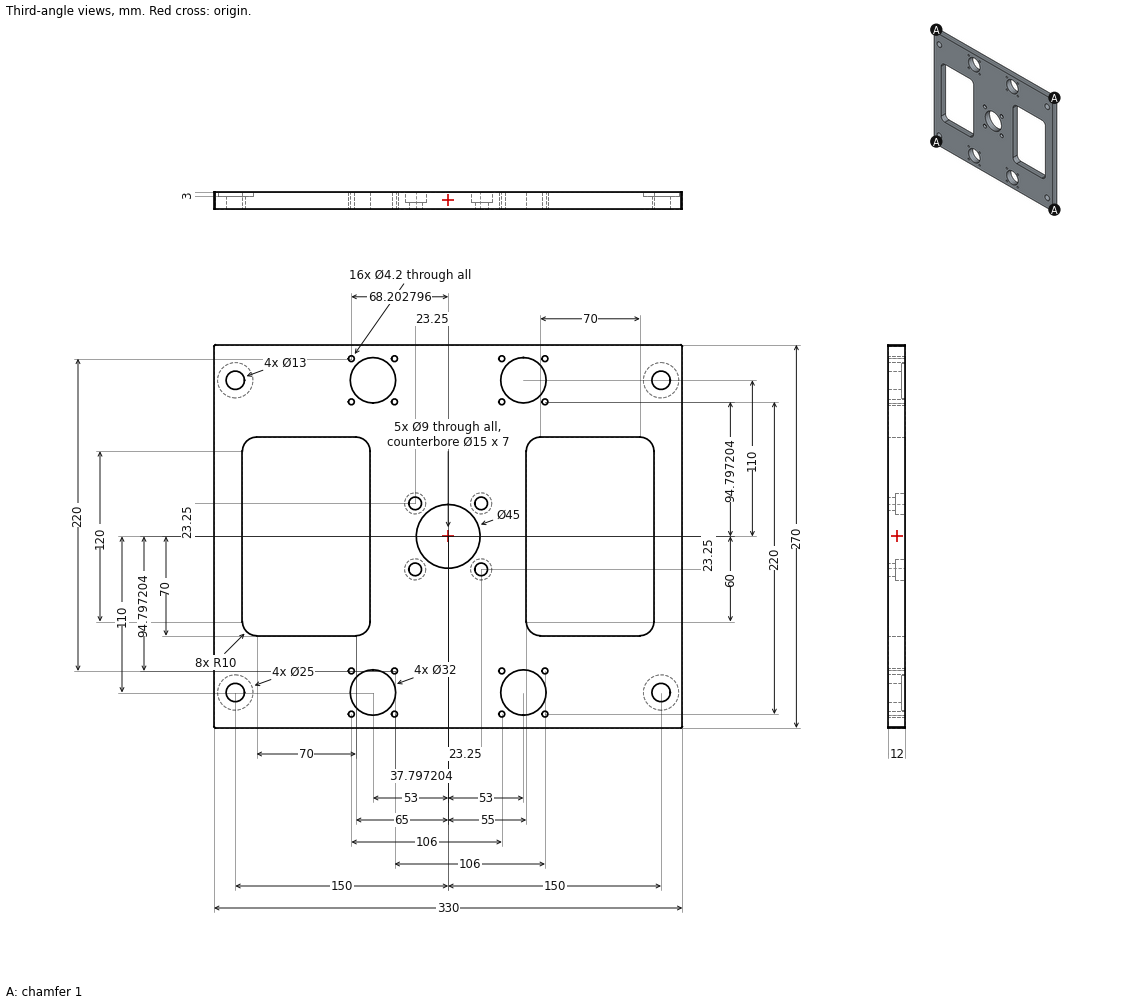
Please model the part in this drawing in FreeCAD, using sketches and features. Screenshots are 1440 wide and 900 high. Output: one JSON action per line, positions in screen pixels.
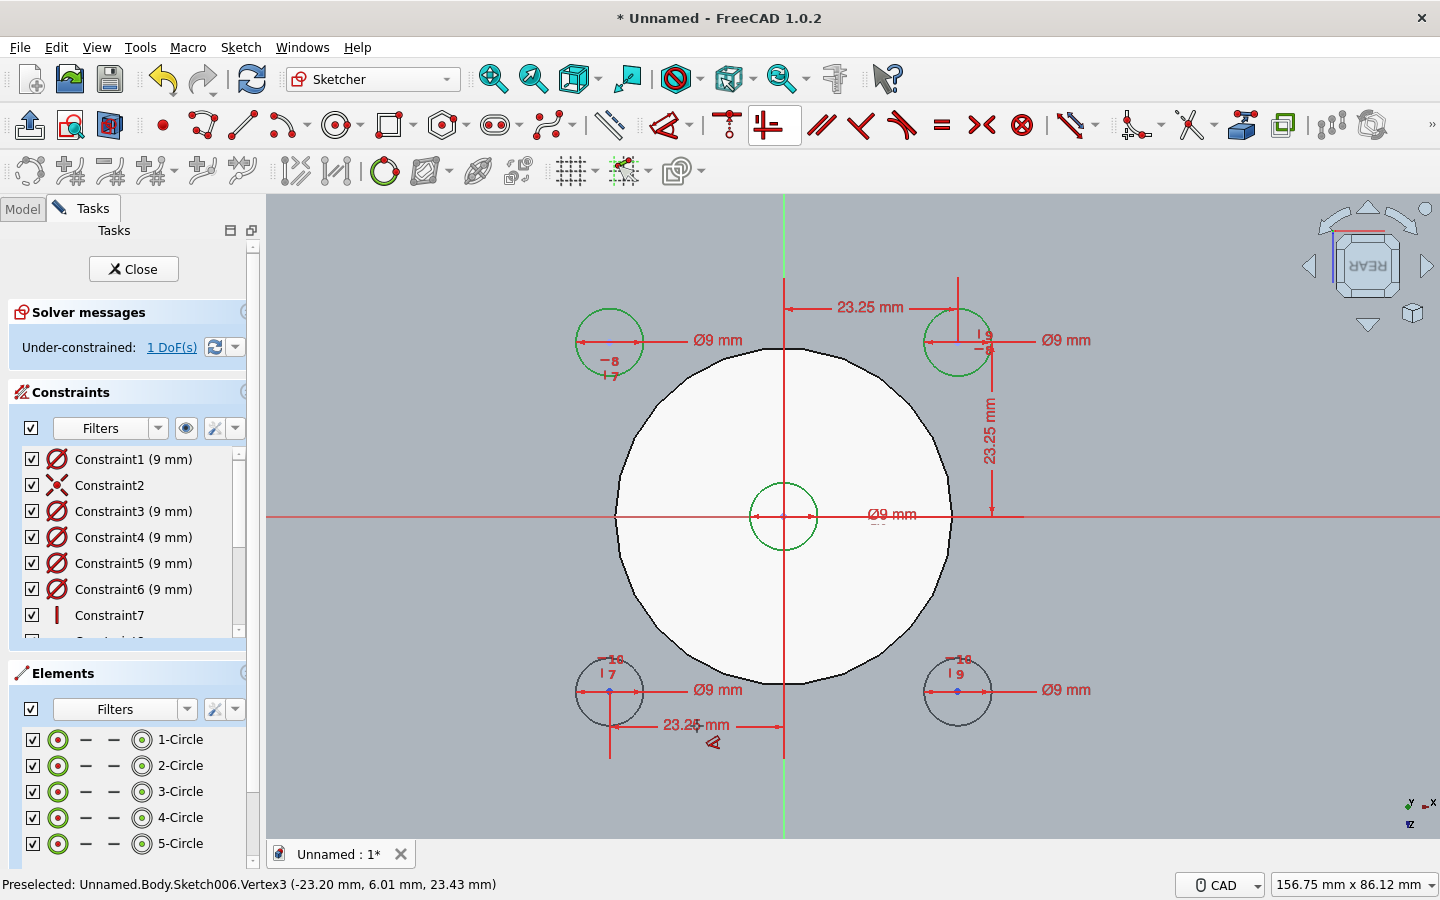
{"action": "left_click", "coordinate": [610, 692]}
{"action": "left_click", "coordinate": [576, 604]}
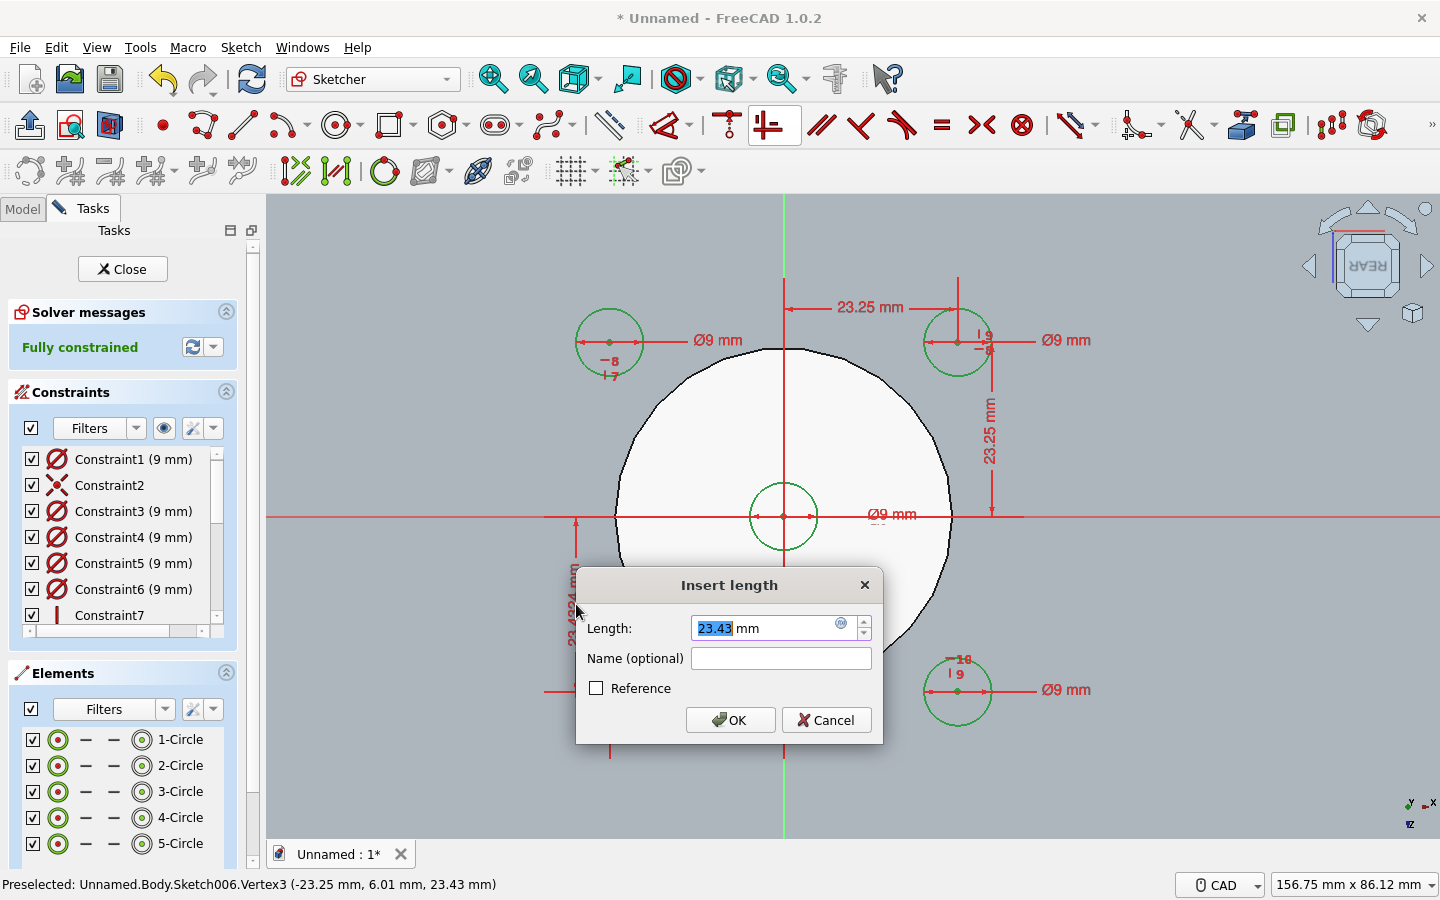
{"action": "type", "text": "23.25"}
{"action": "key", "text": "Return"}
{"action": "key", "text": "Escape"}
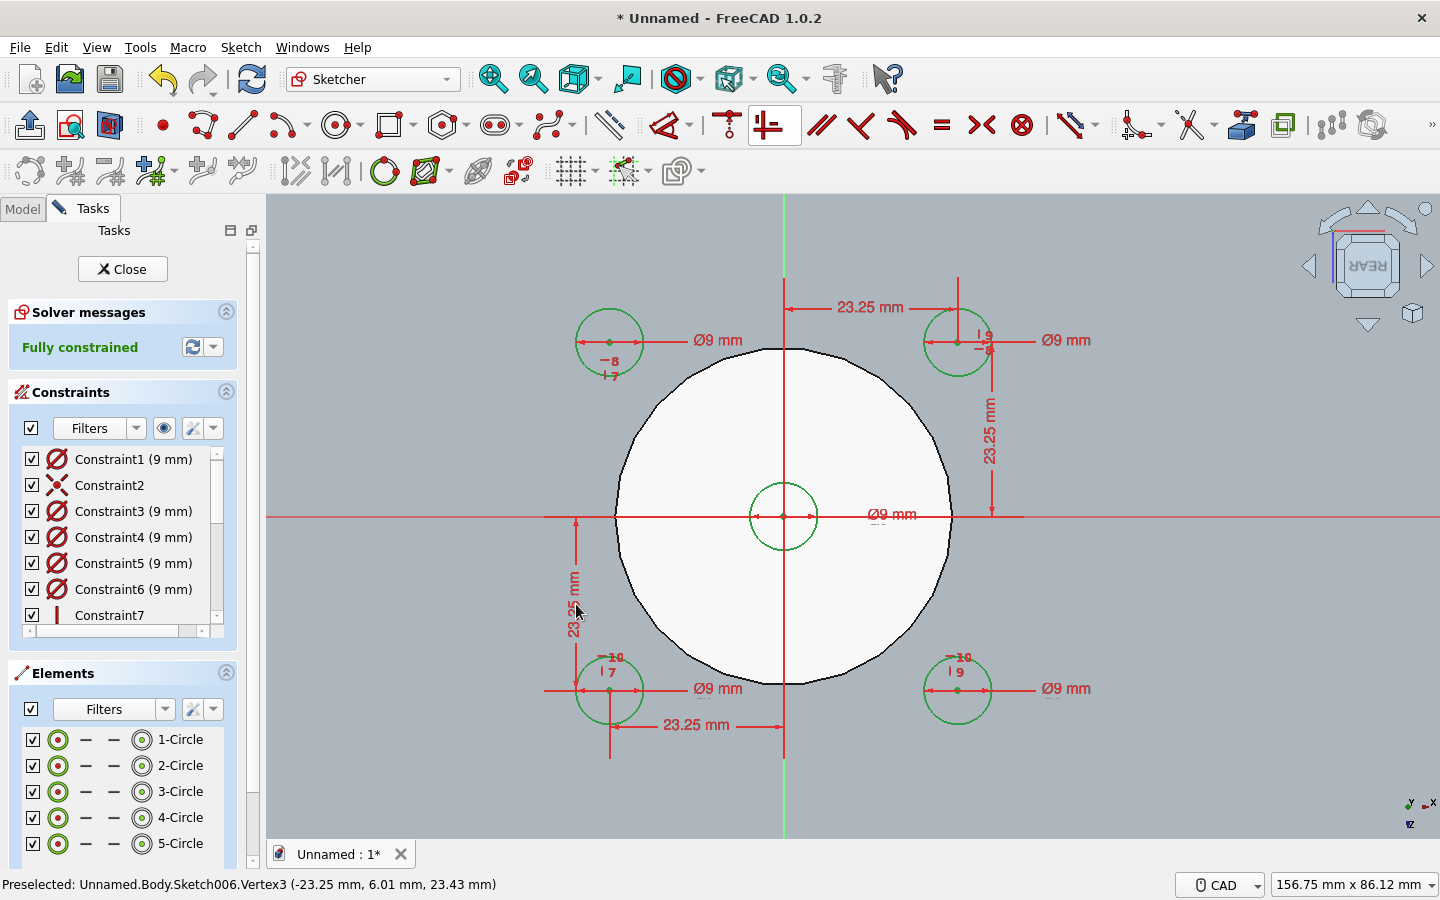
{"action": "left_click", "coordinate": [123, 269]}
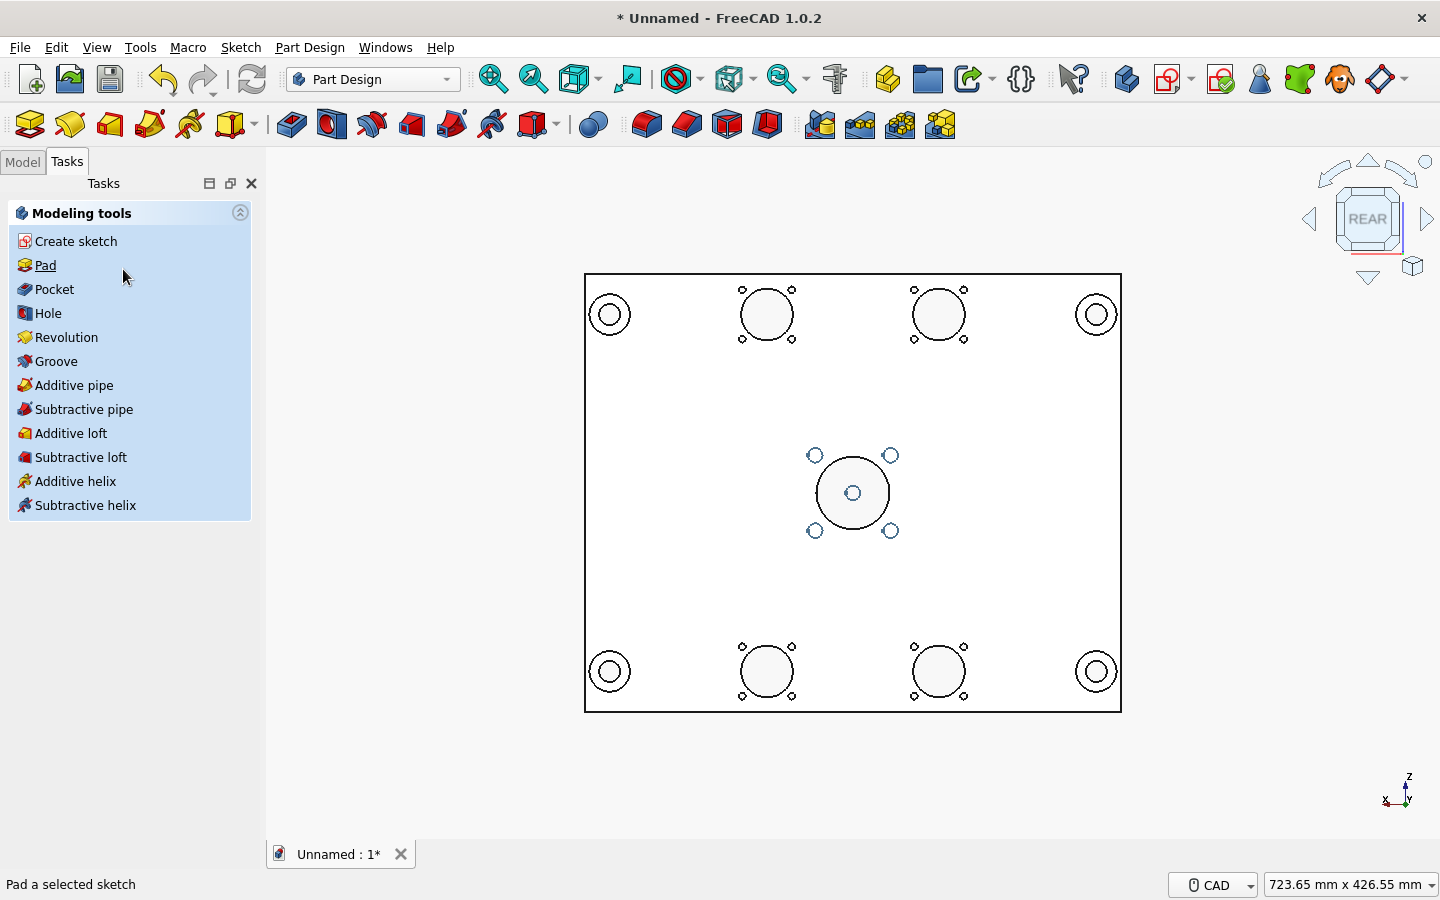
{"action": "left_click", "coordinate": [332, 124]}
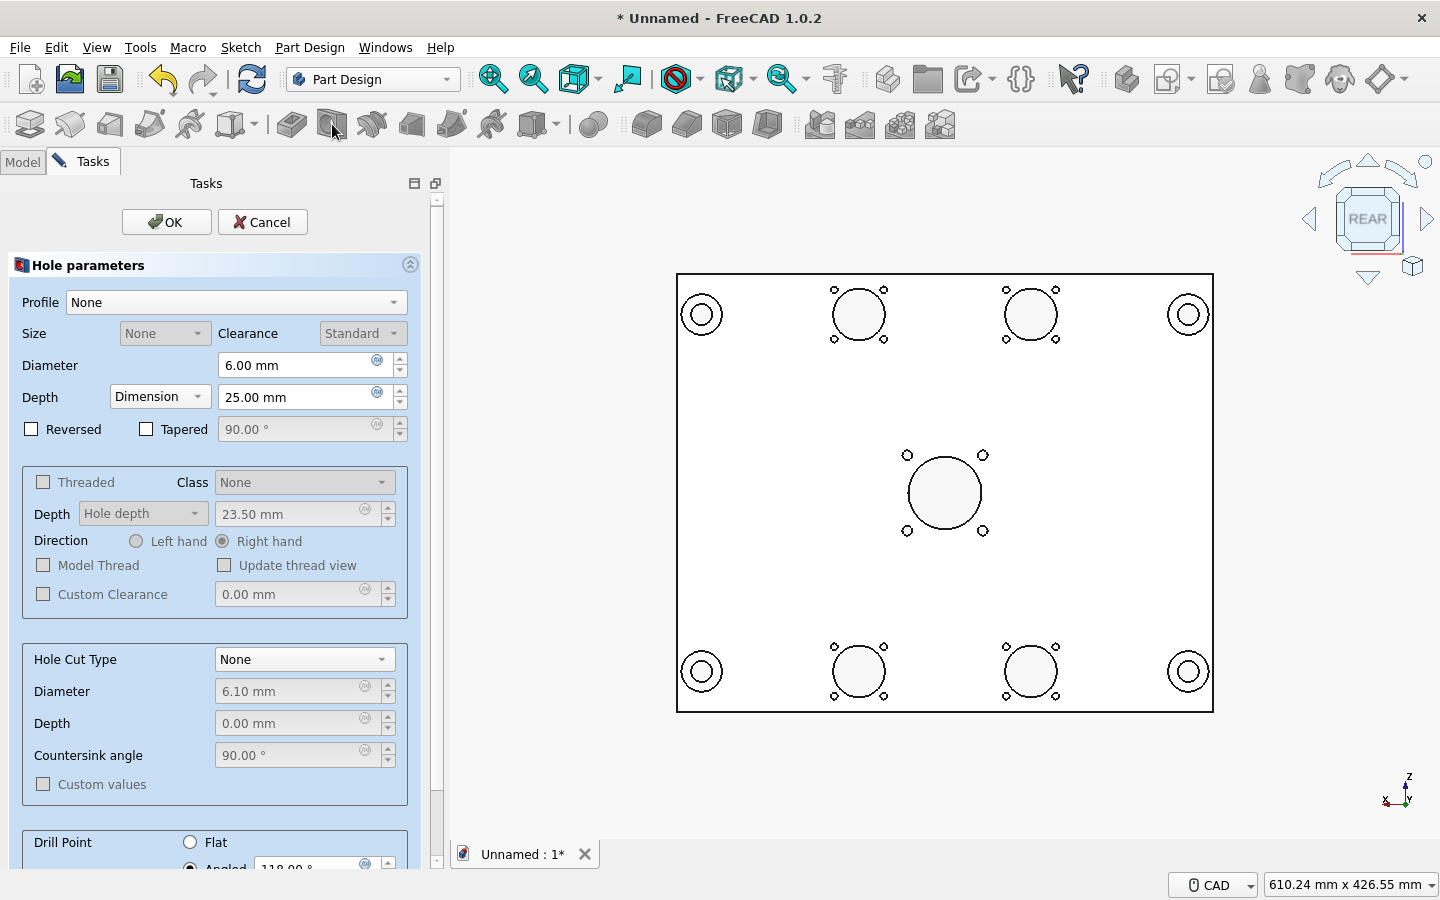
{"action": "triple_click", "coordinate": [305, 365]}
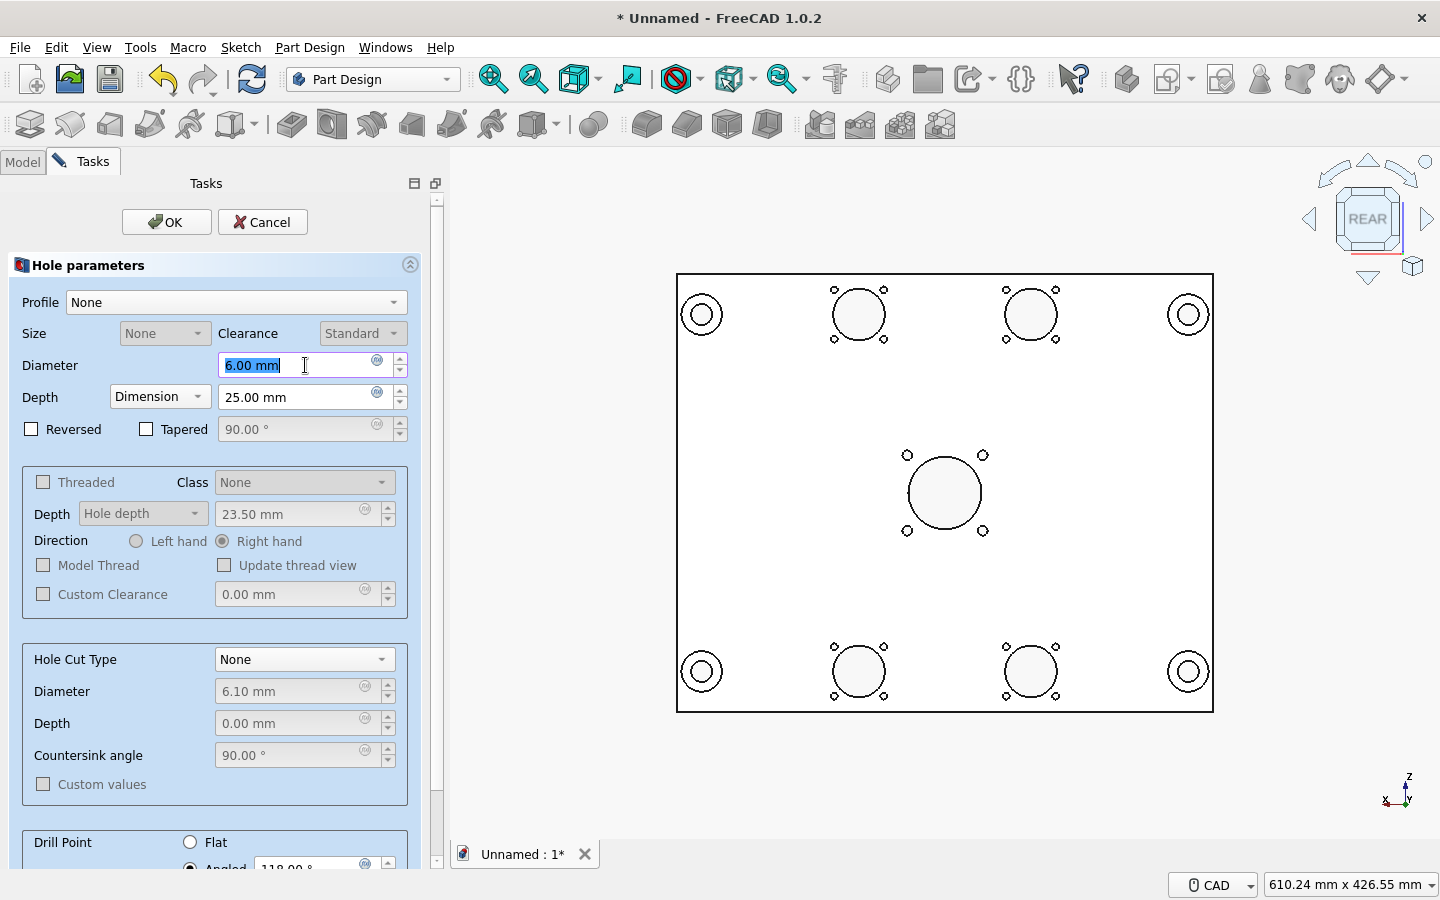
{"action": "type", "text": "9"}
{"action": "key", "text": "Tab"}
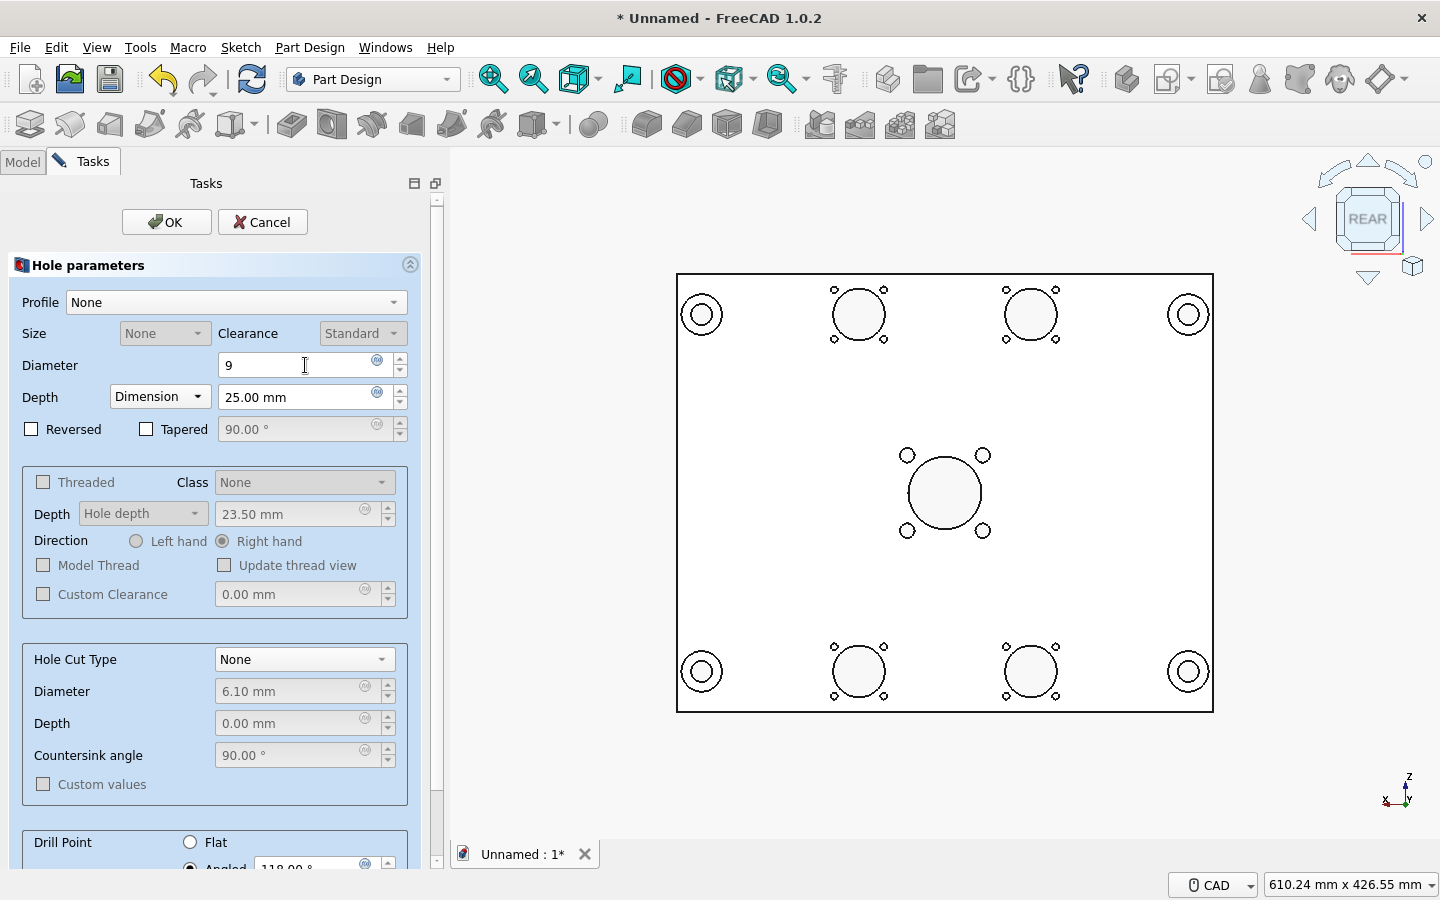
{"action": "left_click", "coordinate": [161, 396]}